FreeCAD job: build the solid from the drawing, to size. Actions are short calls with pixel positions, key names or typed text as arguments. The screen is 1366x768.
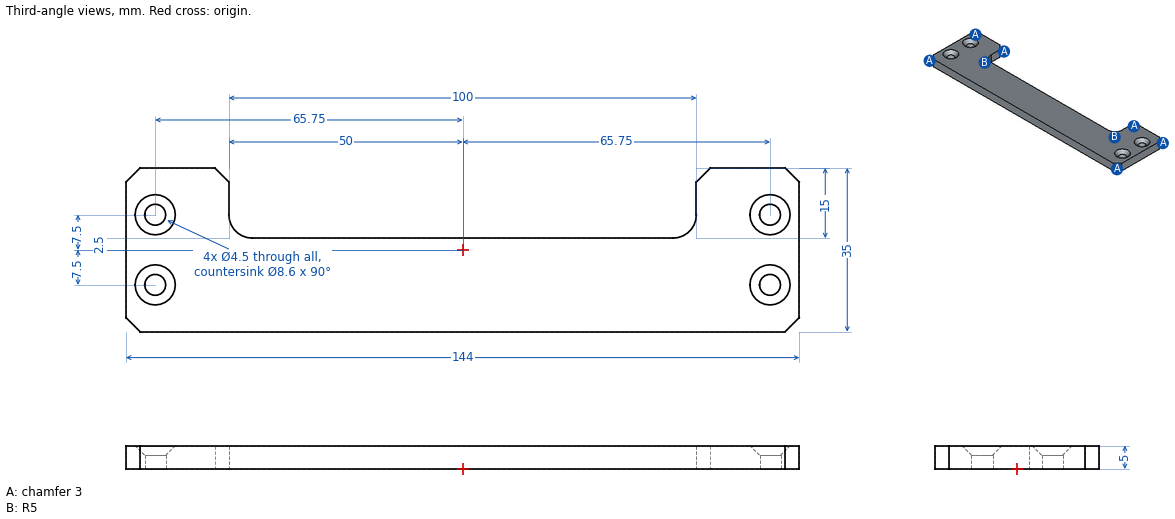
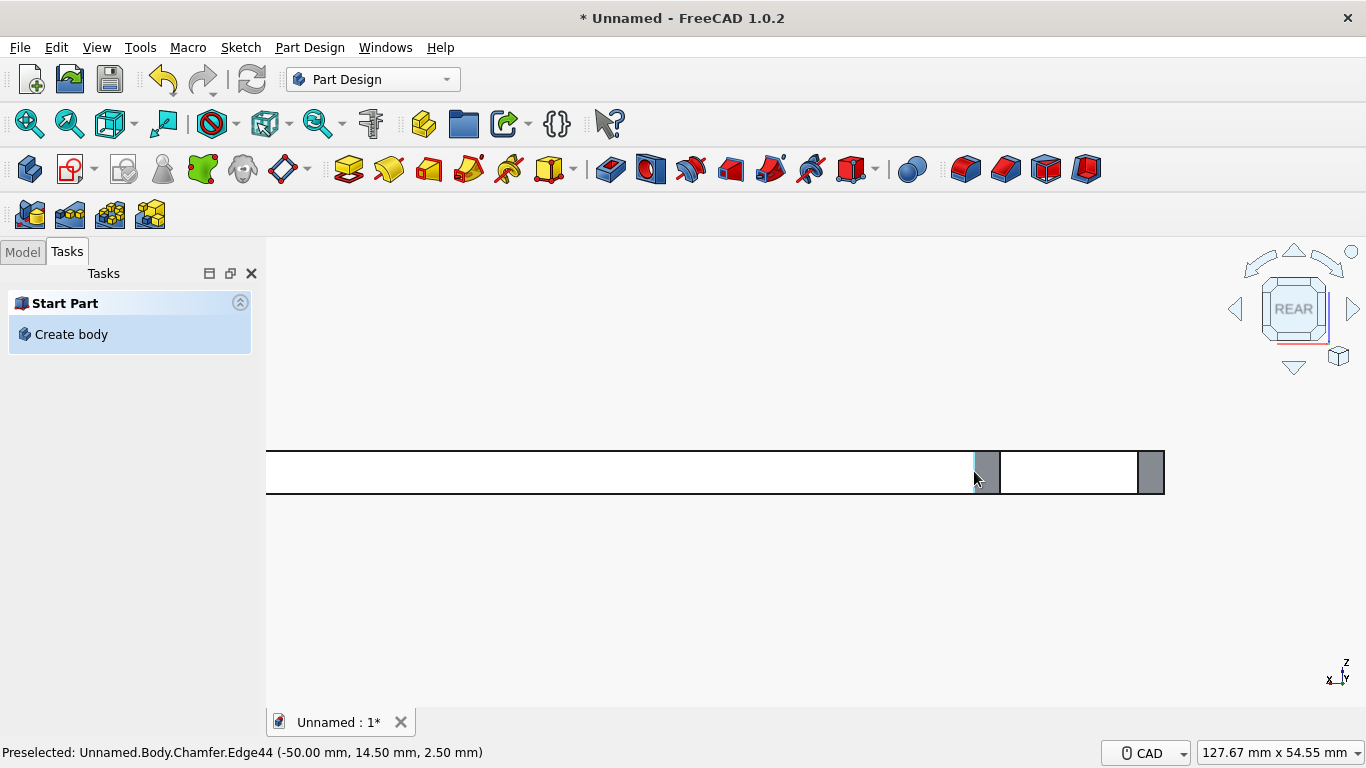
key(v)
key(f)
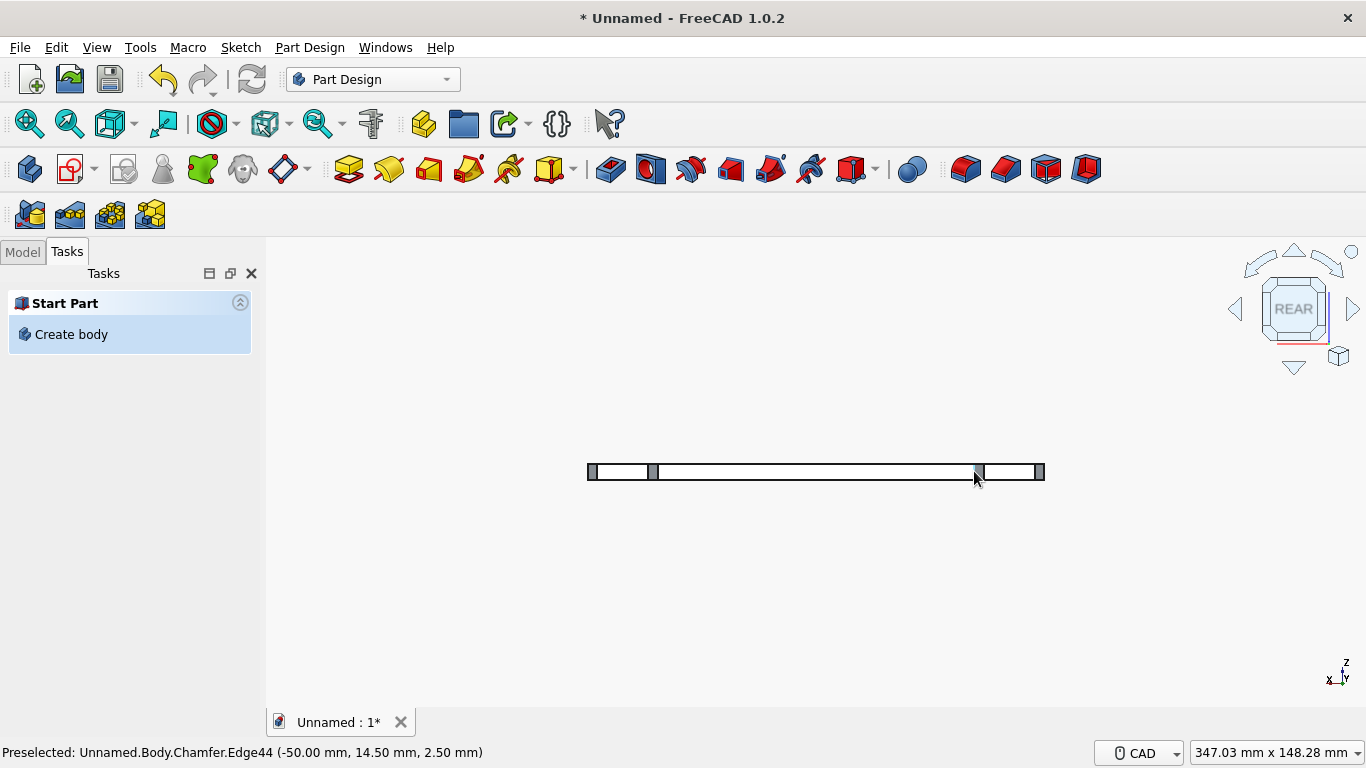
key(6)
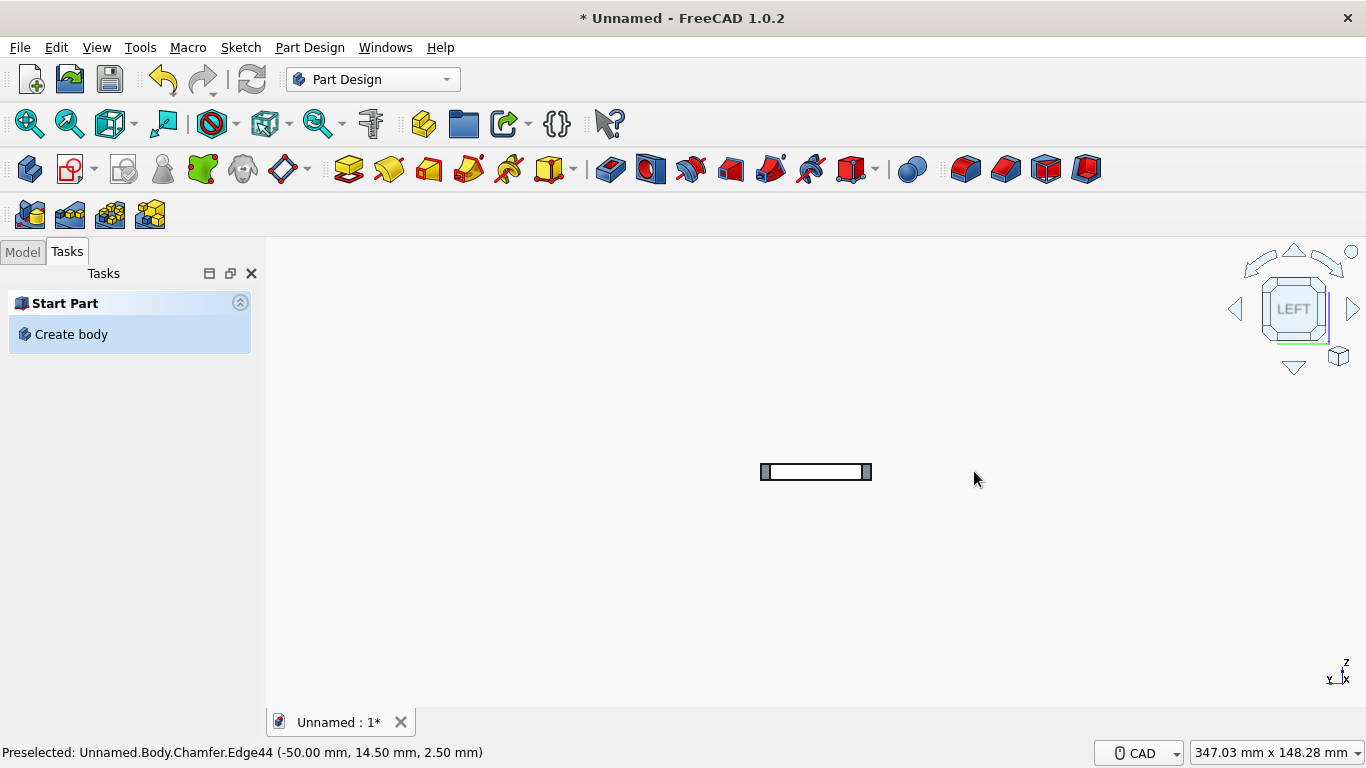
key(v)
key(f)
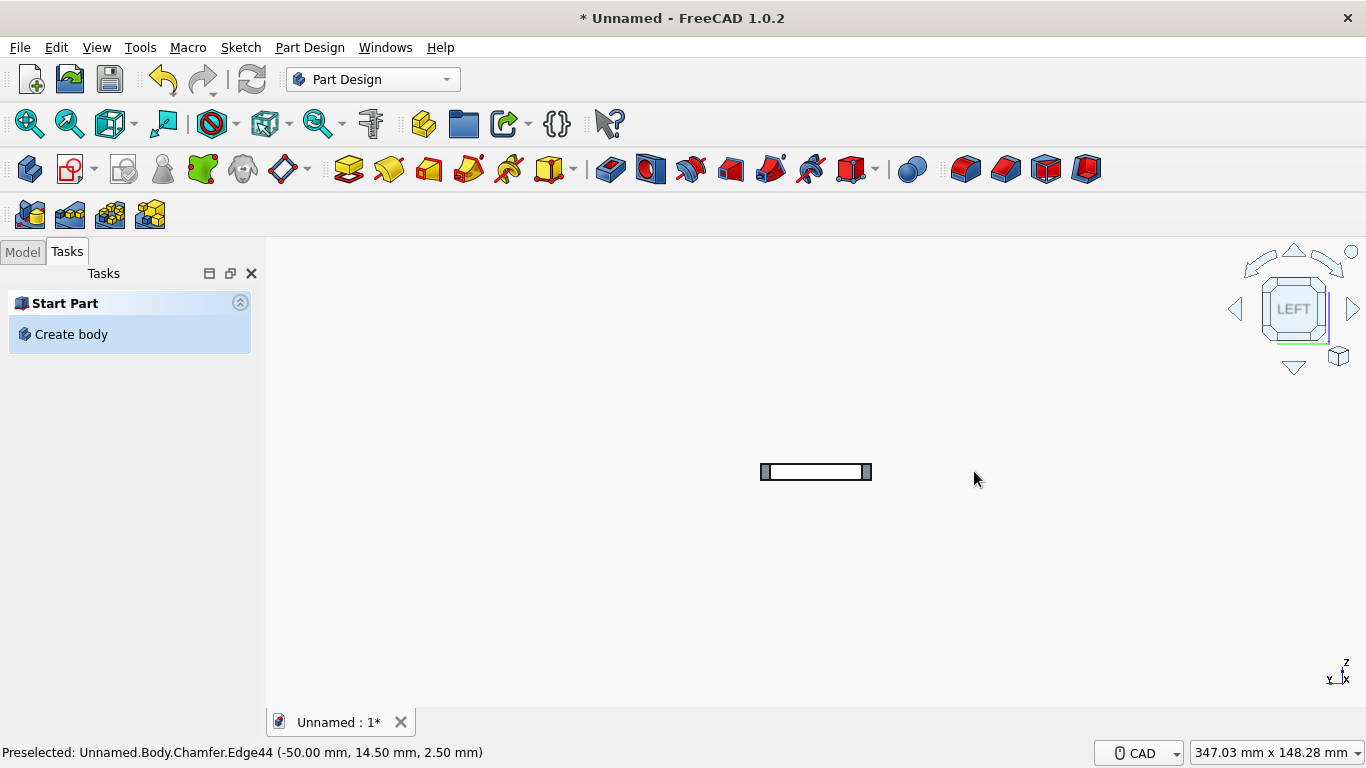
scroll(808, 471, up, 5)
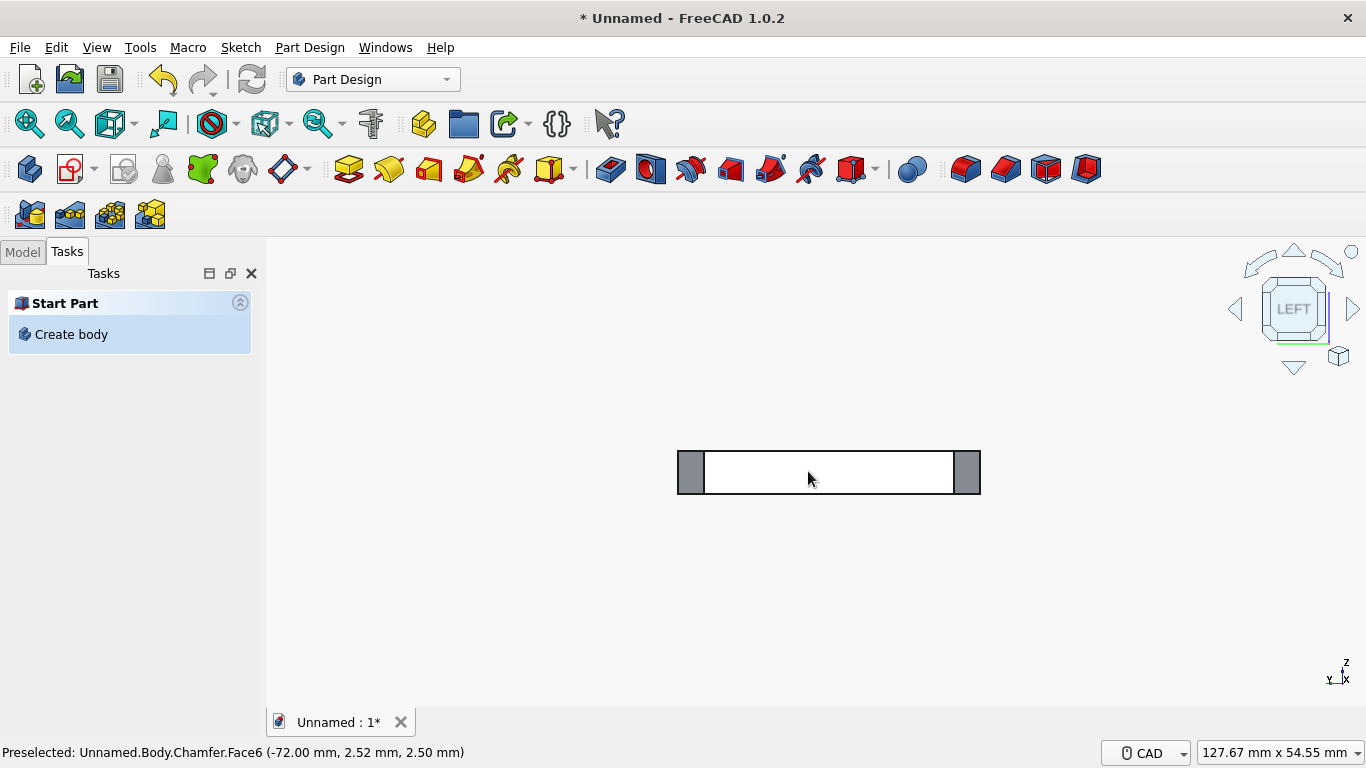
key(v)
key(f)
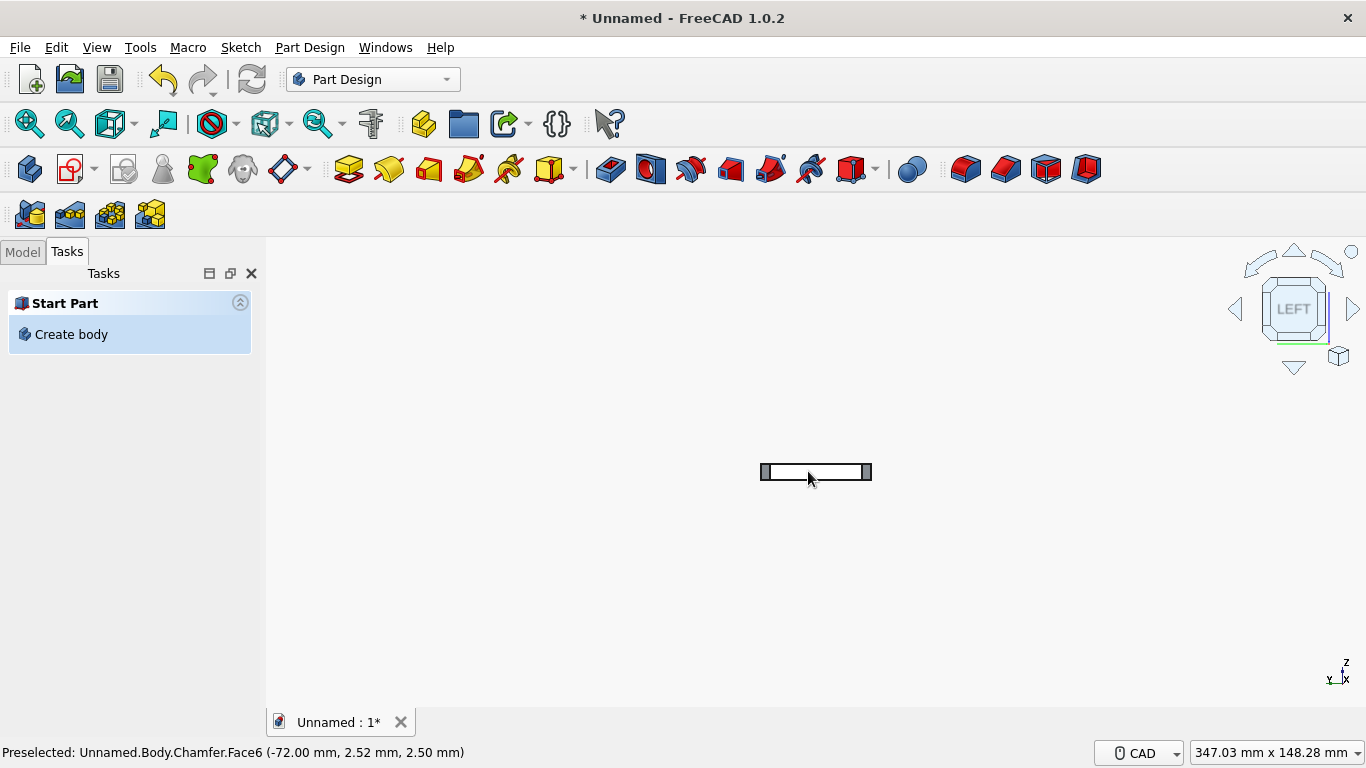
key(v)
key(3)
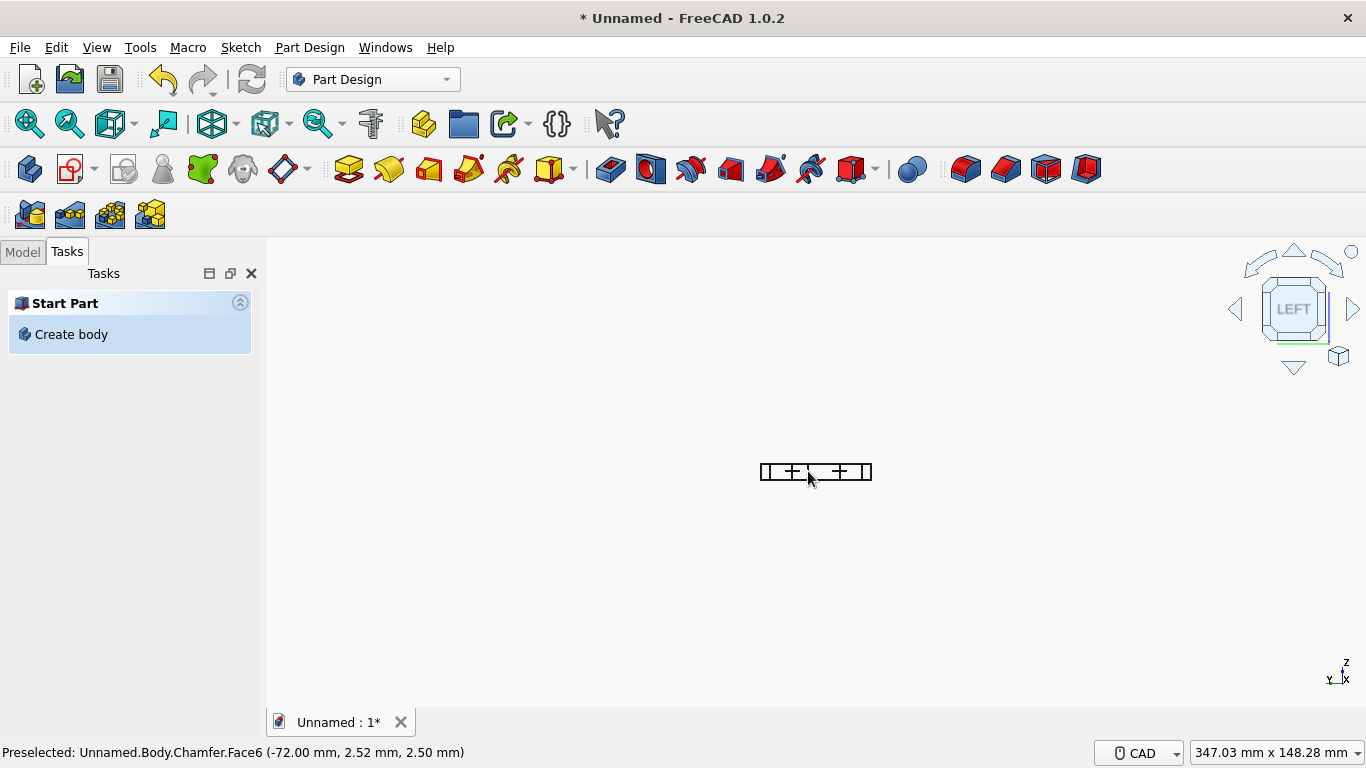
key(0)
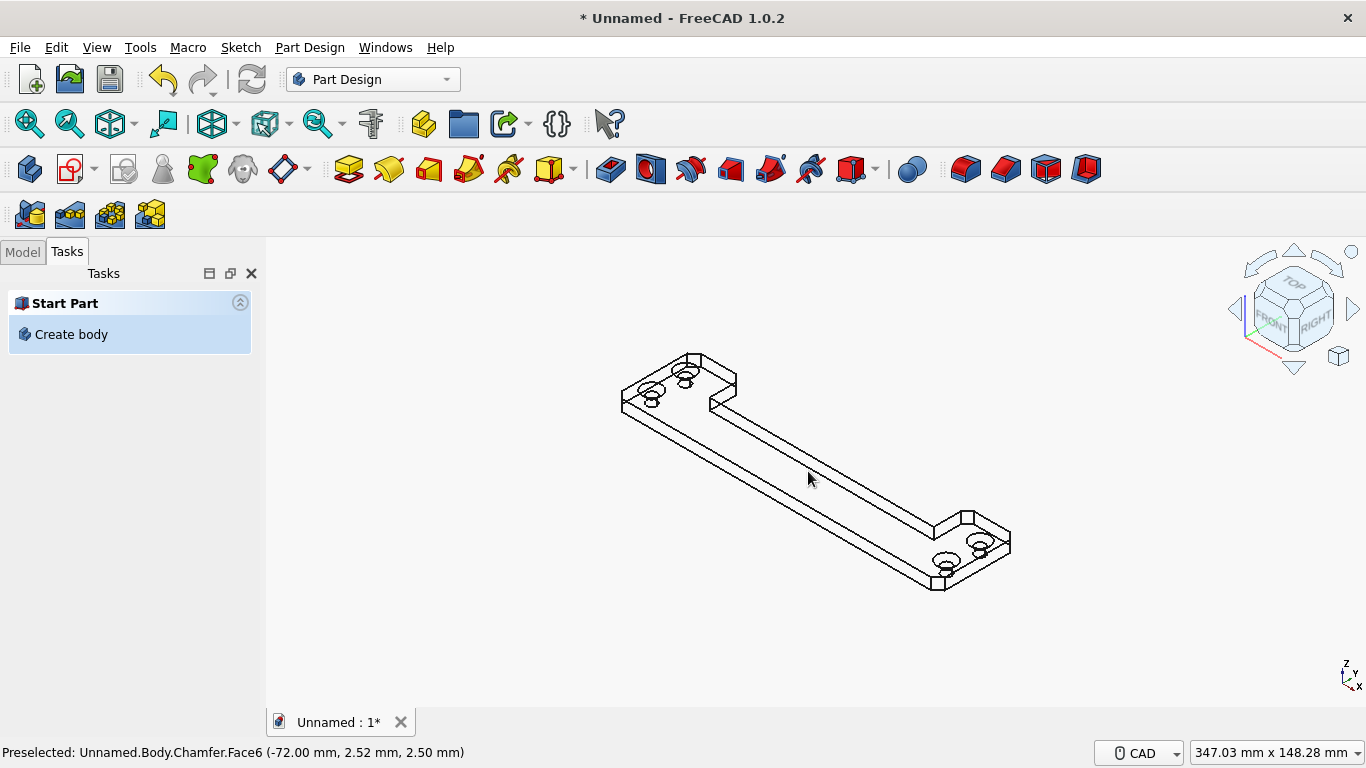
click(710, 406)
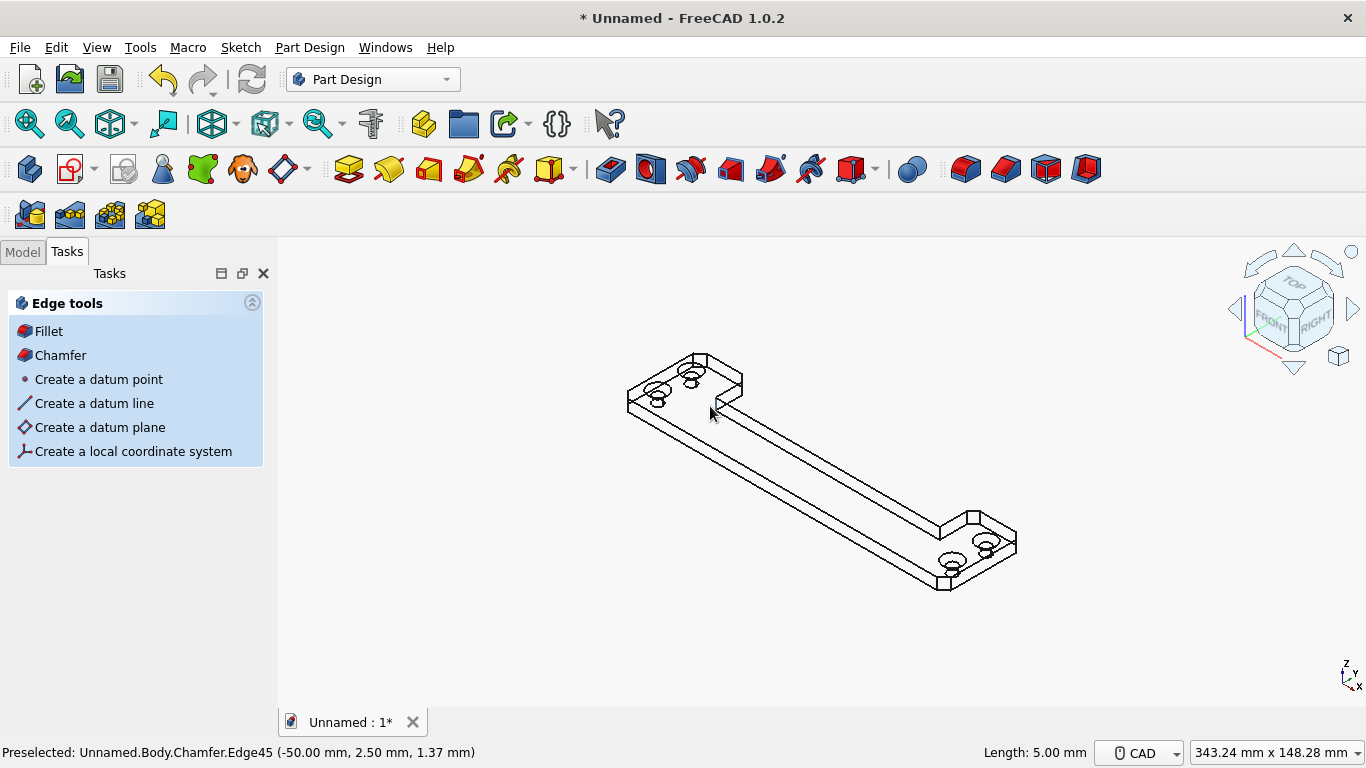
click(940, 532, ctrl)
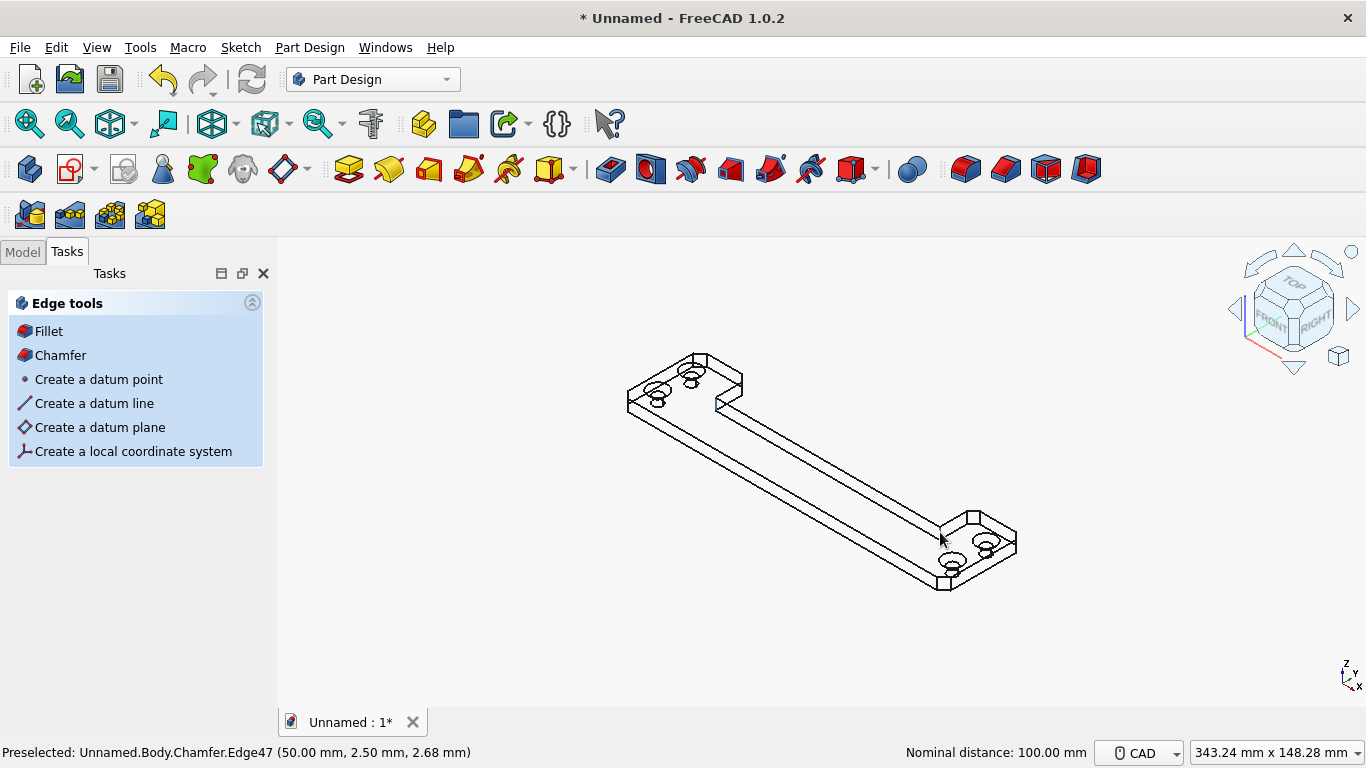
key(v)
key(1)